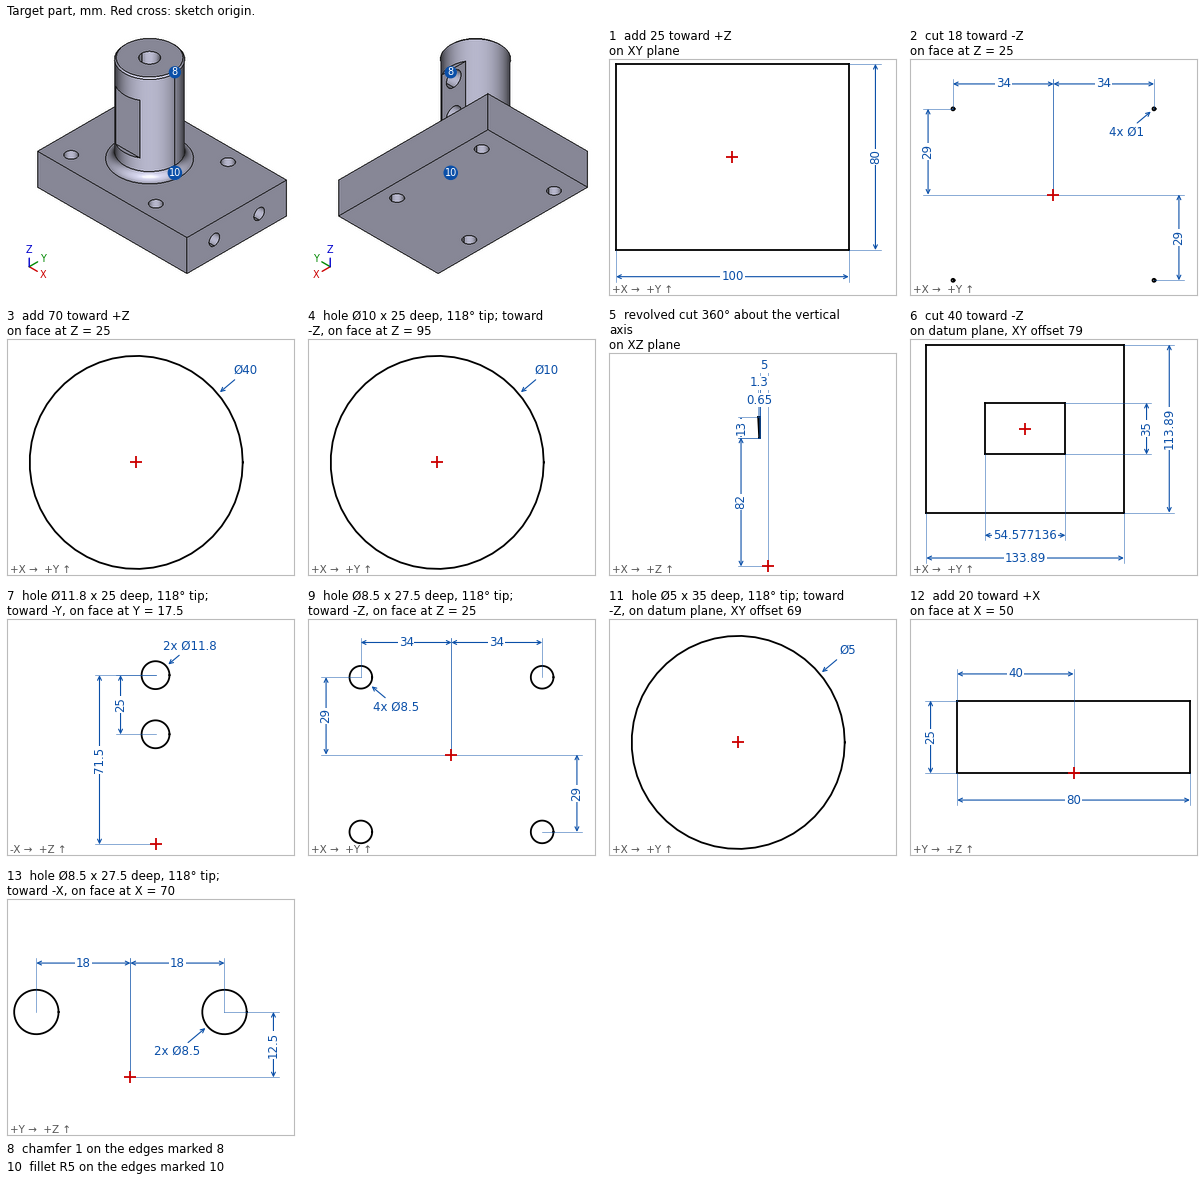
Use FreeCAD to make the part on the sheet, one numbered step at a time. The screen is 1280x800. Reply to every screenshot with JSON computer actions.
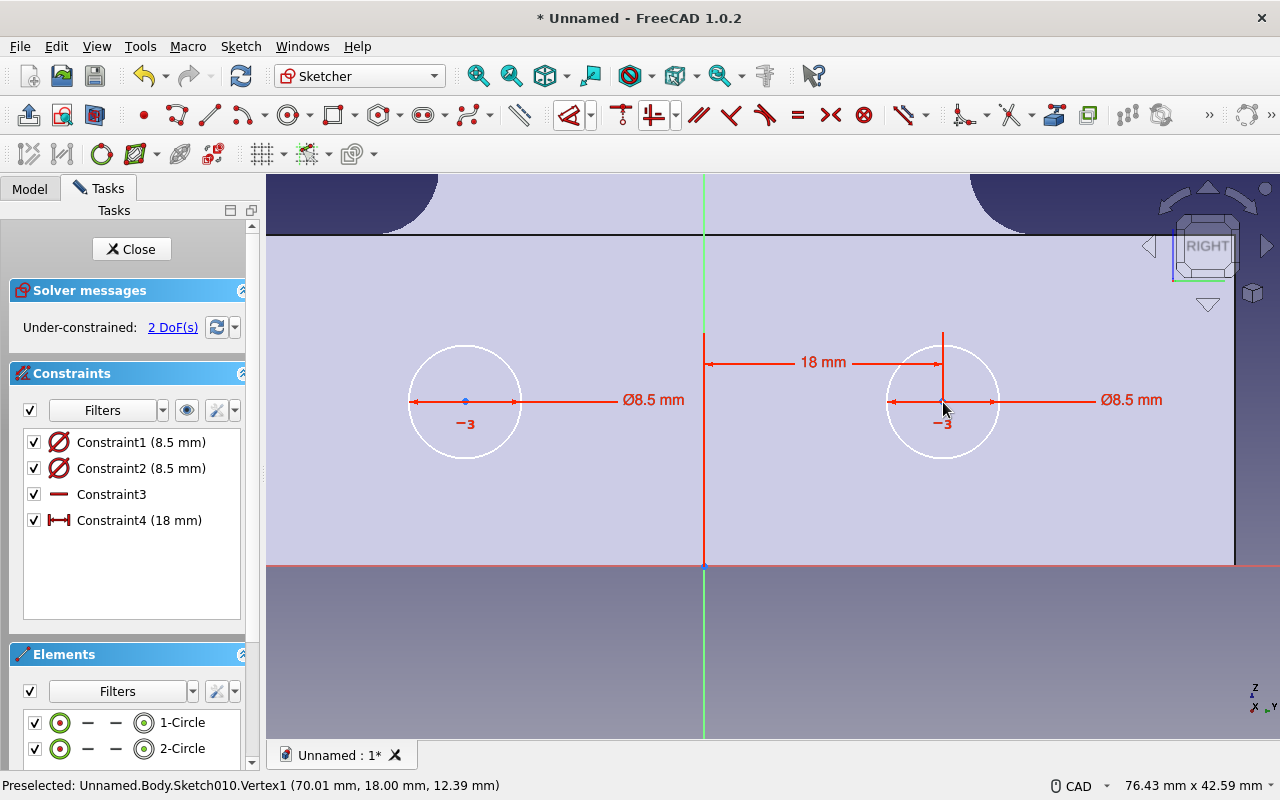
{"action": "left_click", "coordinate": [465, 402]}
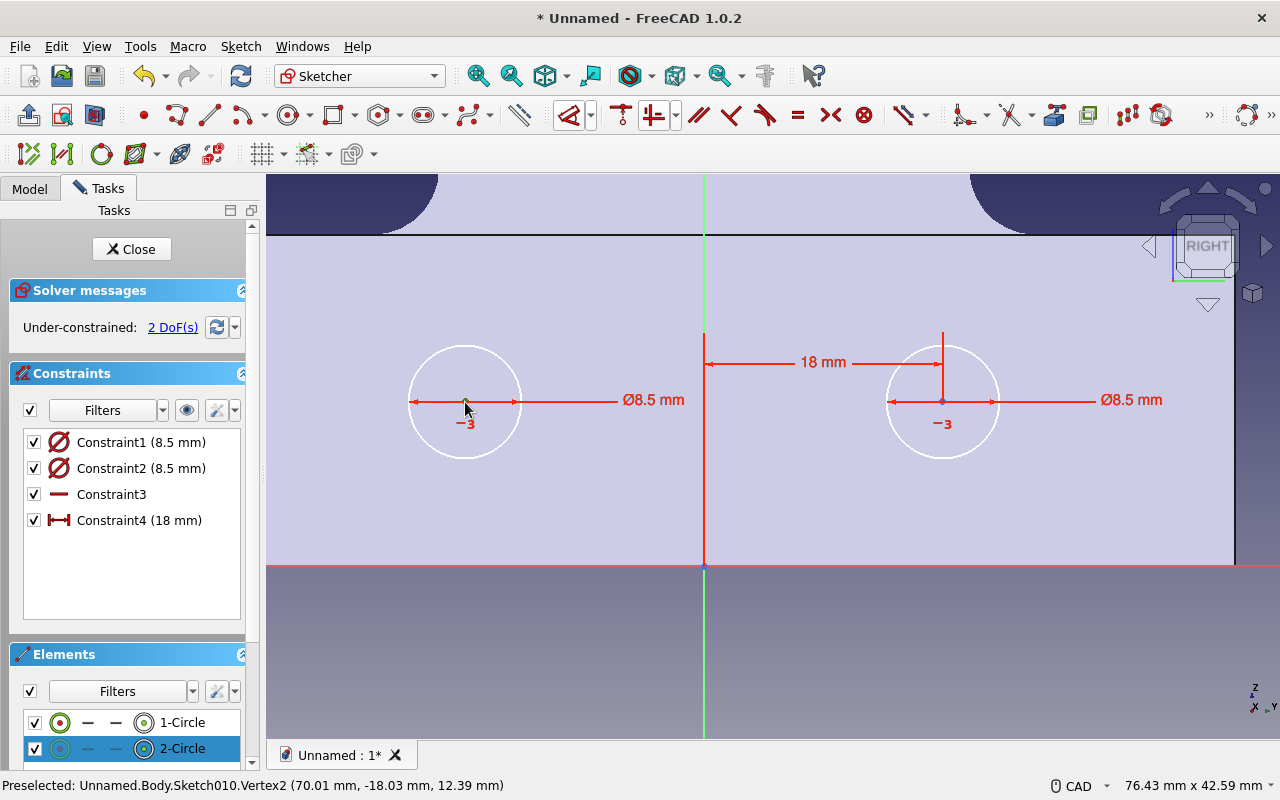
{"action": "key", "text": "l"}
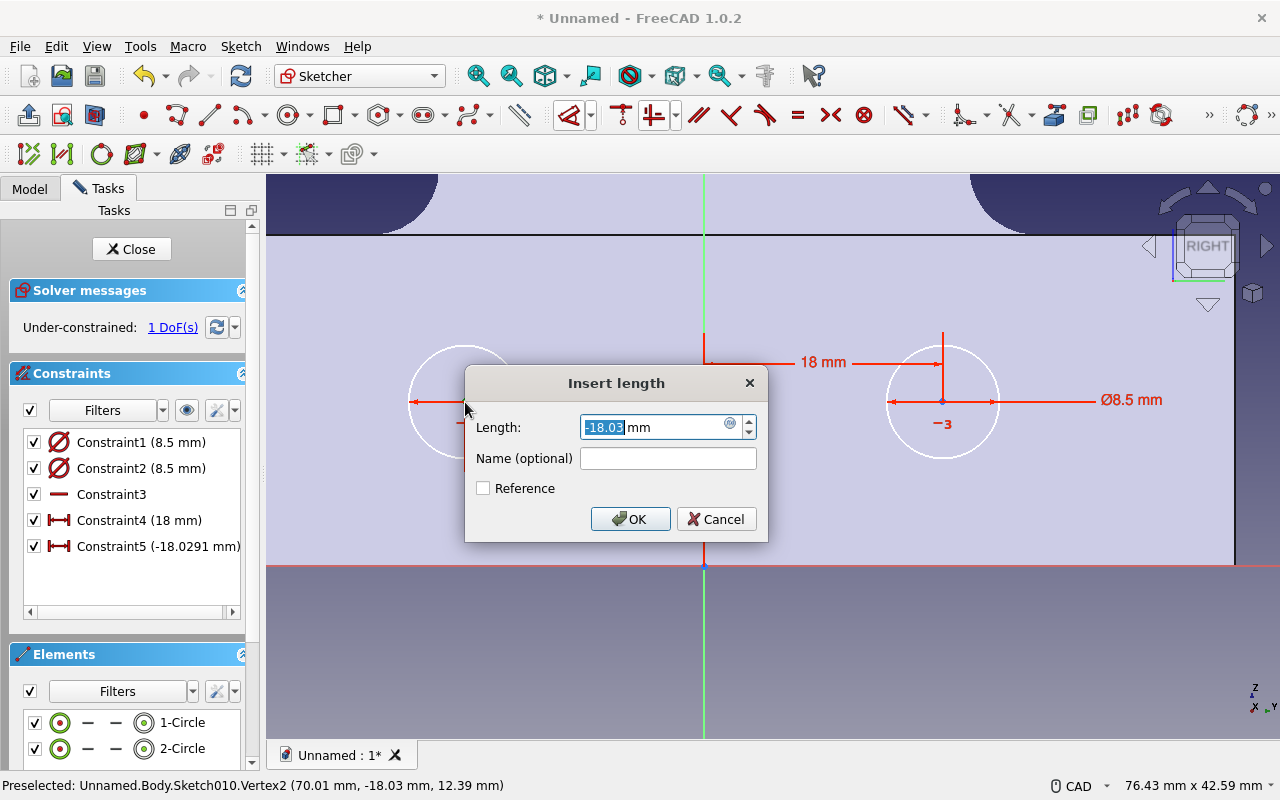
{"action": "type", "text": "-18"}
{"action": "key", "text": "Return"}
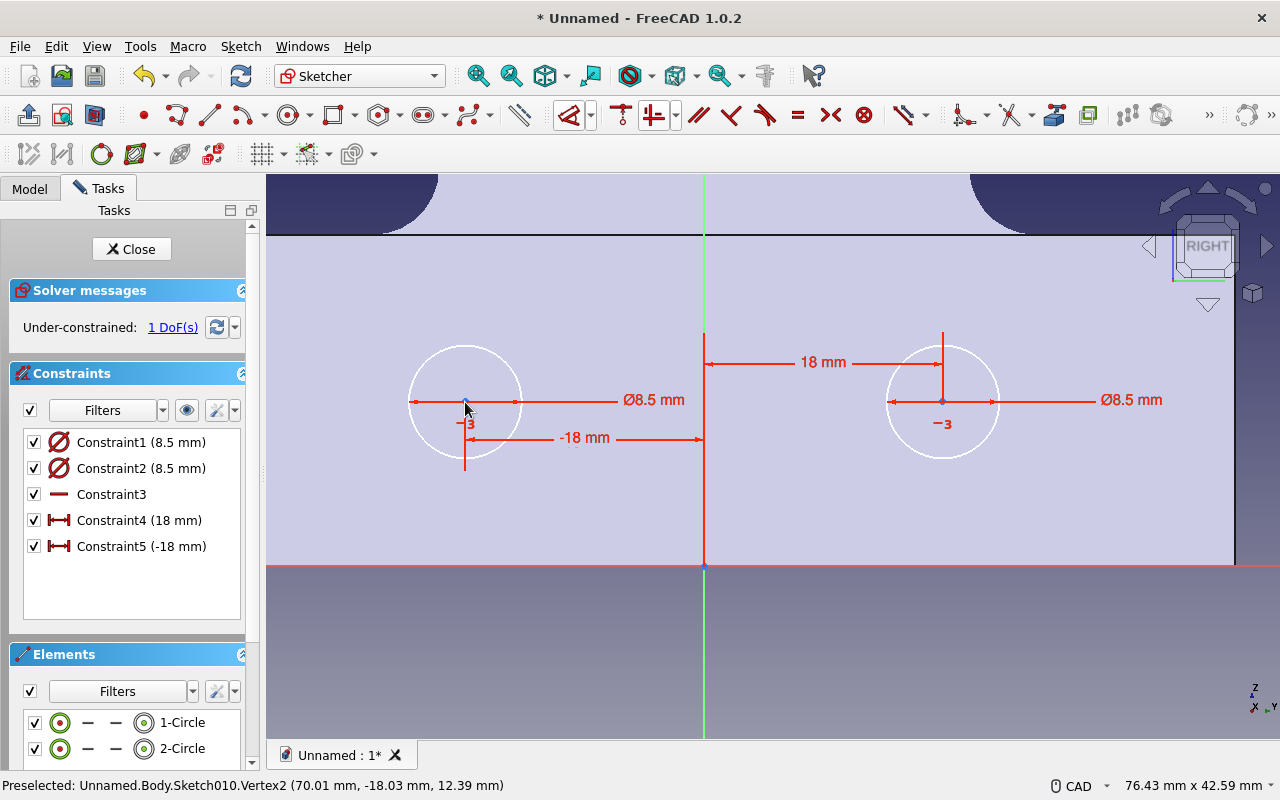
{"action": "left_click", "coordinate": [943, 402]}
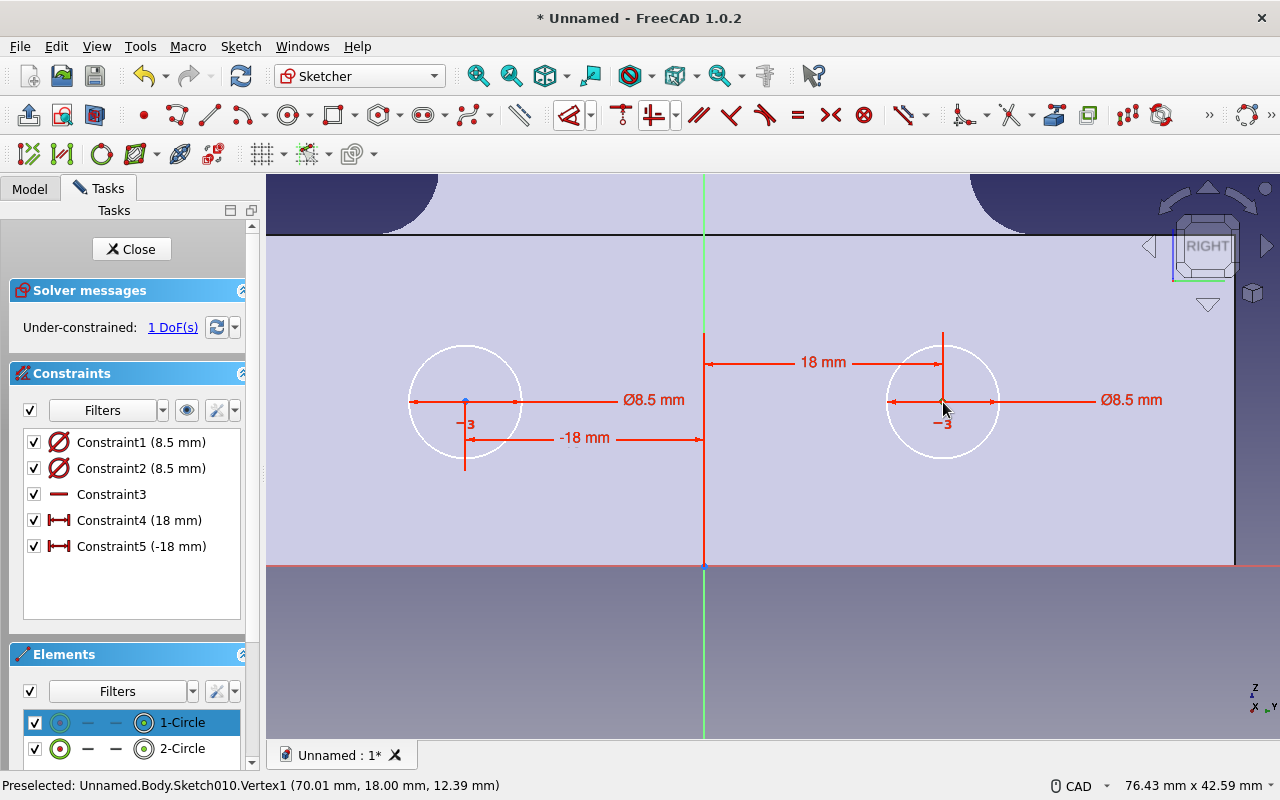
{"action": "key", "text": "i"}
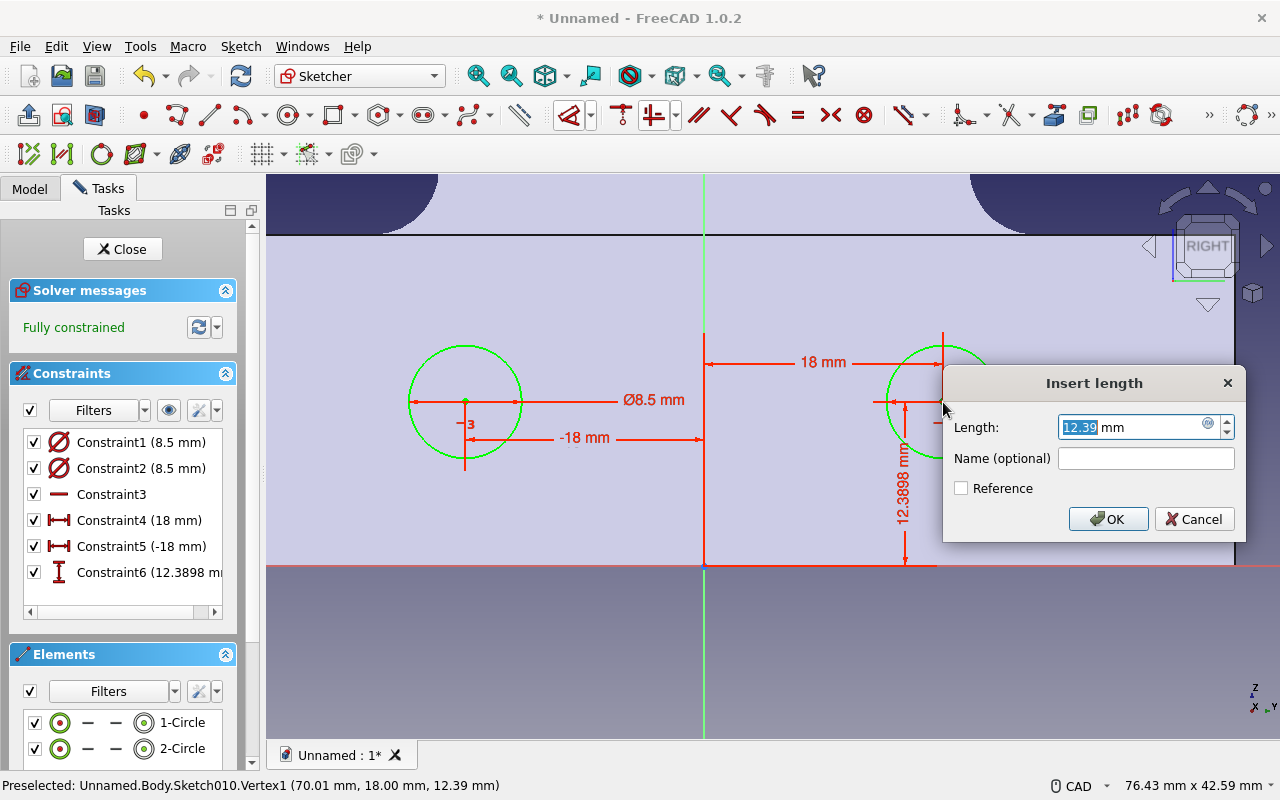
{"action": "type", "text": "12.5"}
{"action": "key", "text": "Return"}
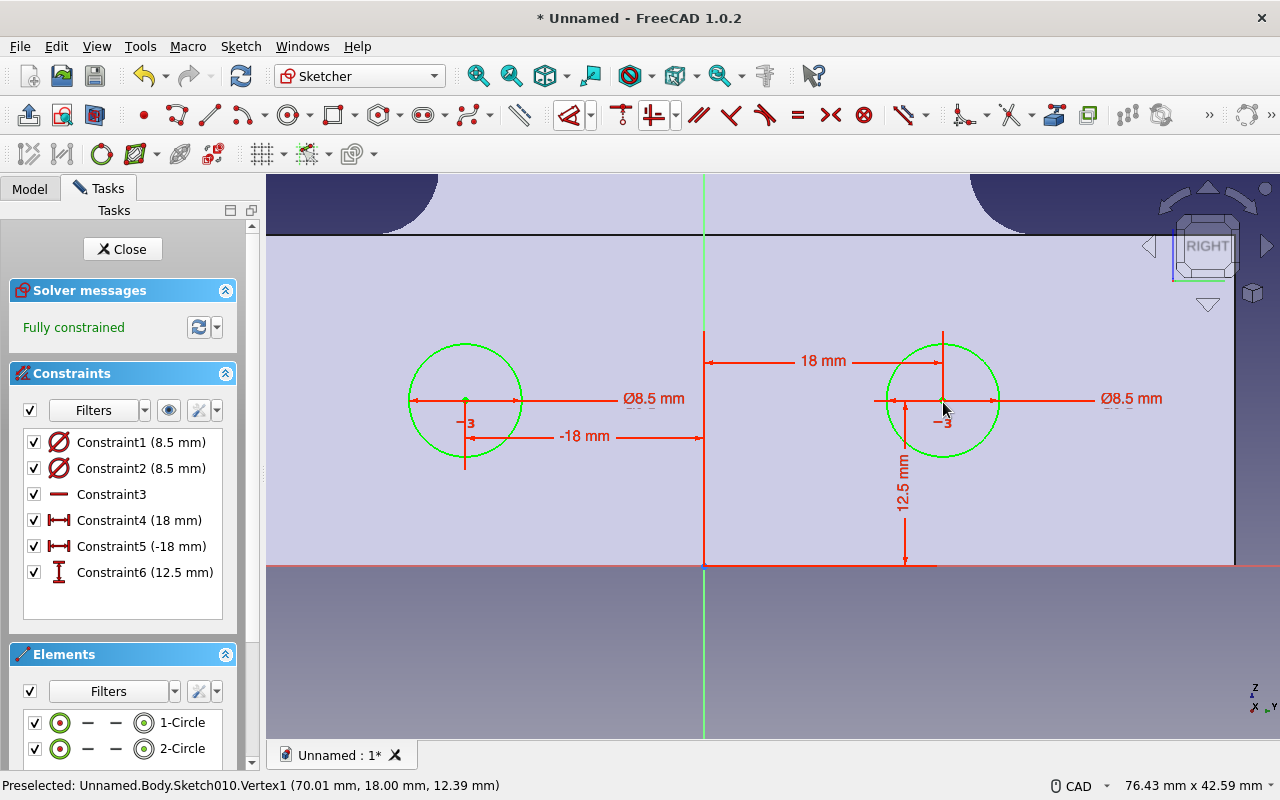
{"action": "left_click", "coordinate": [123, 249]}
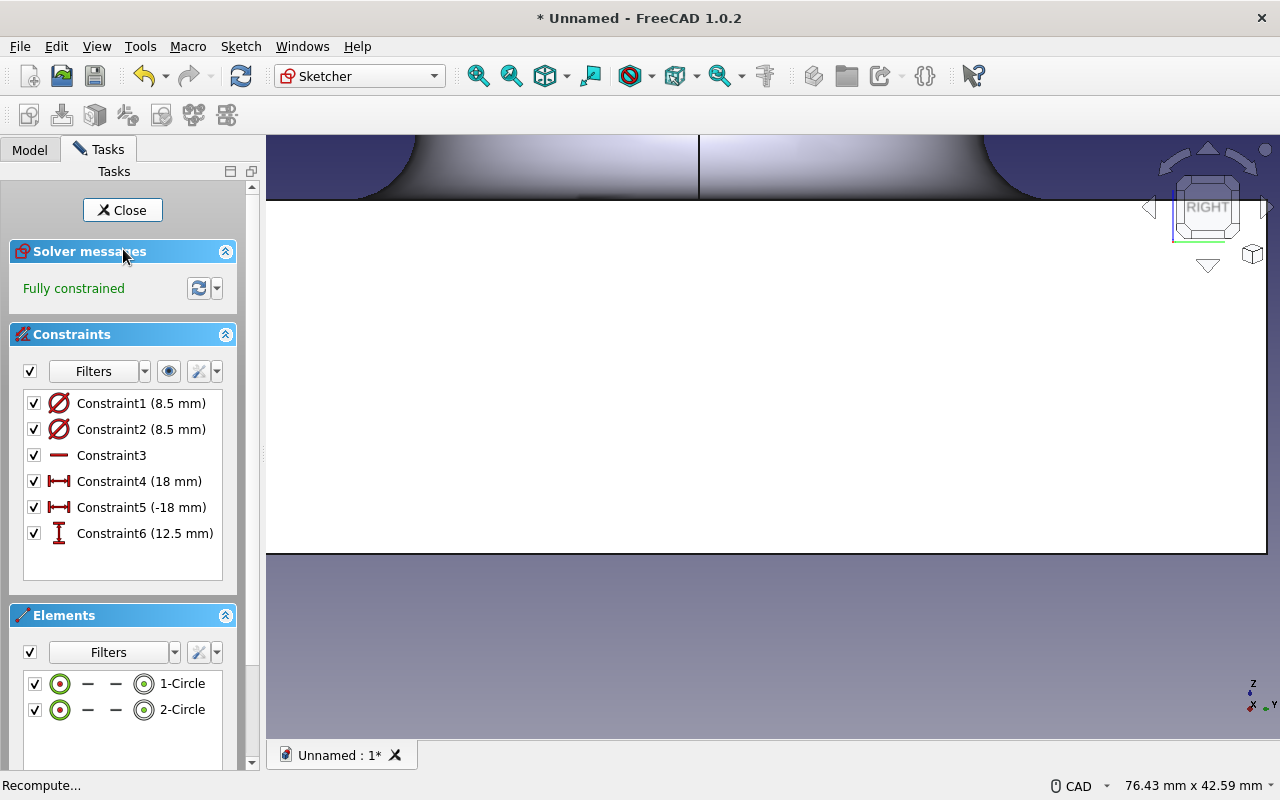
{"action": "left_click", "coordinate": [279, 116]}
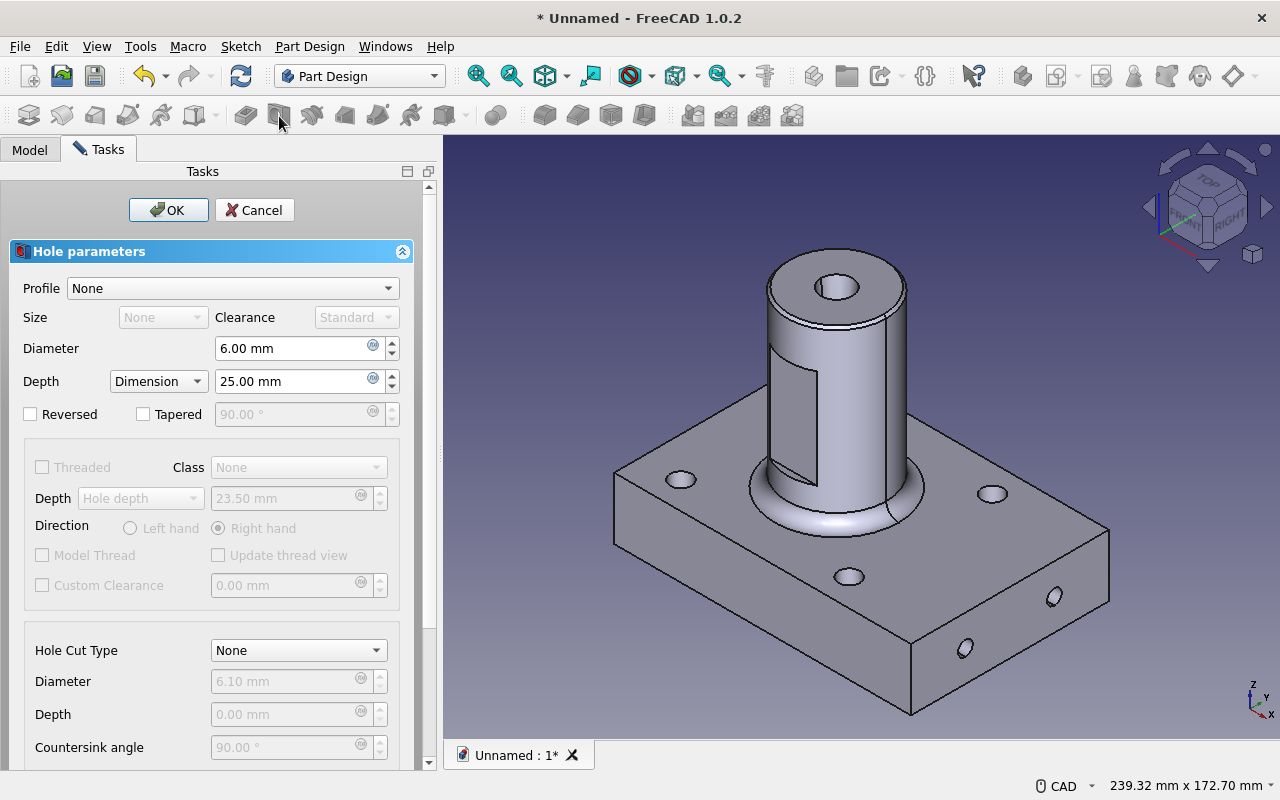
{"action": "triple_click", "coordinate": [300, 348]}